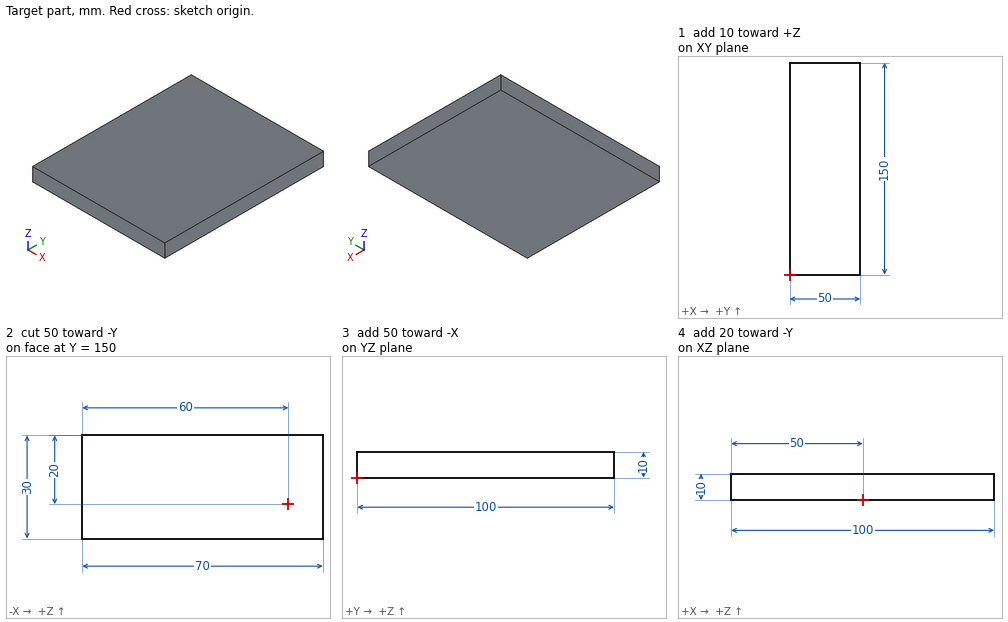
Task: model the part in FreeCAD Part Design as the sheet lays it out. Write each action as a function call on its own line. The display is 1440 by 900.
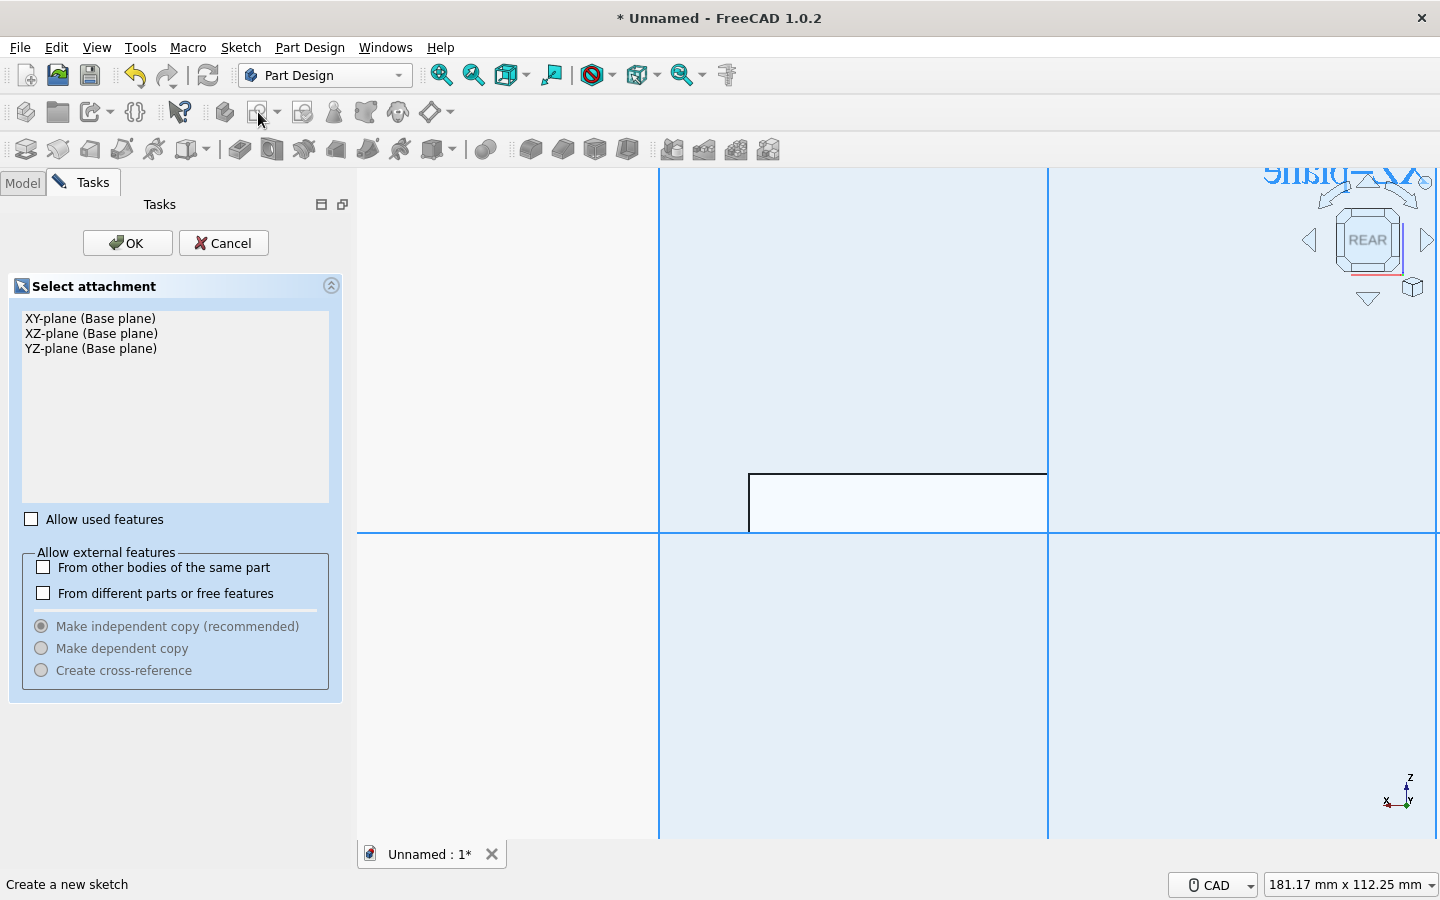
click(82, 348)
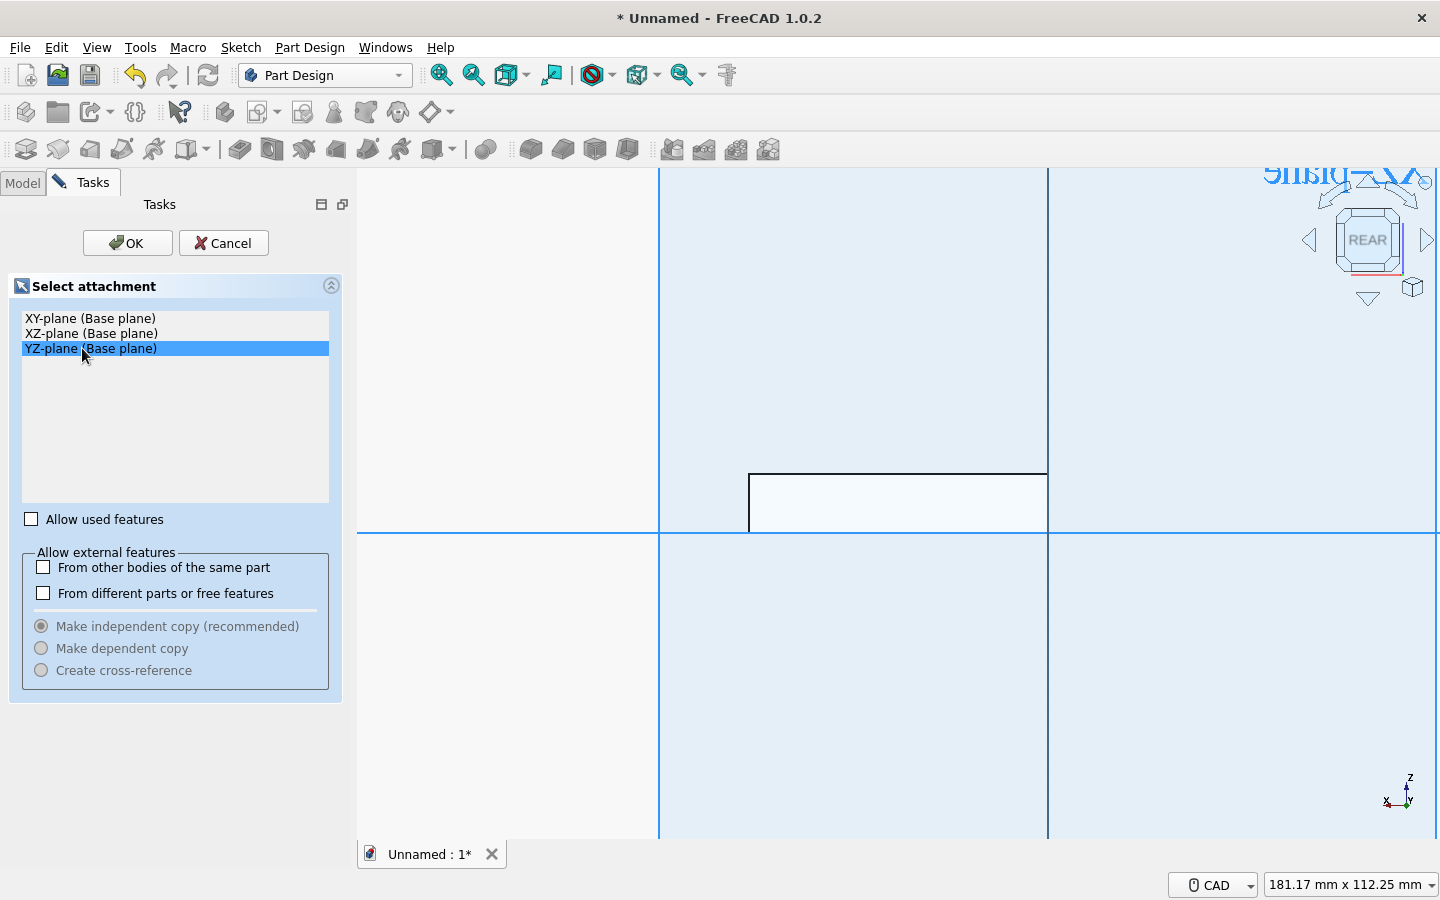
click(128, 243)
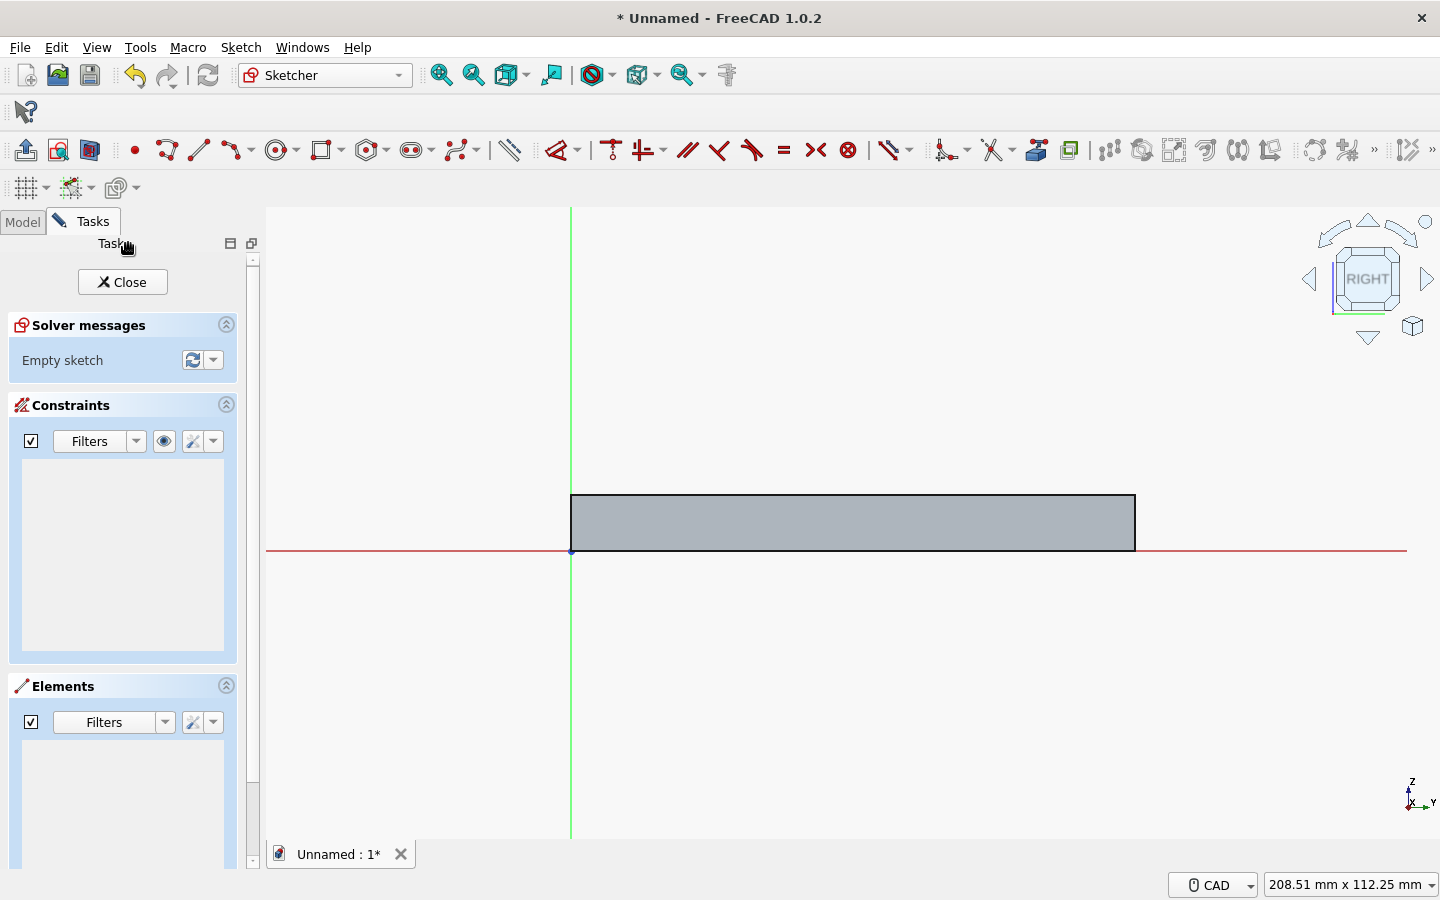
click(90, 150)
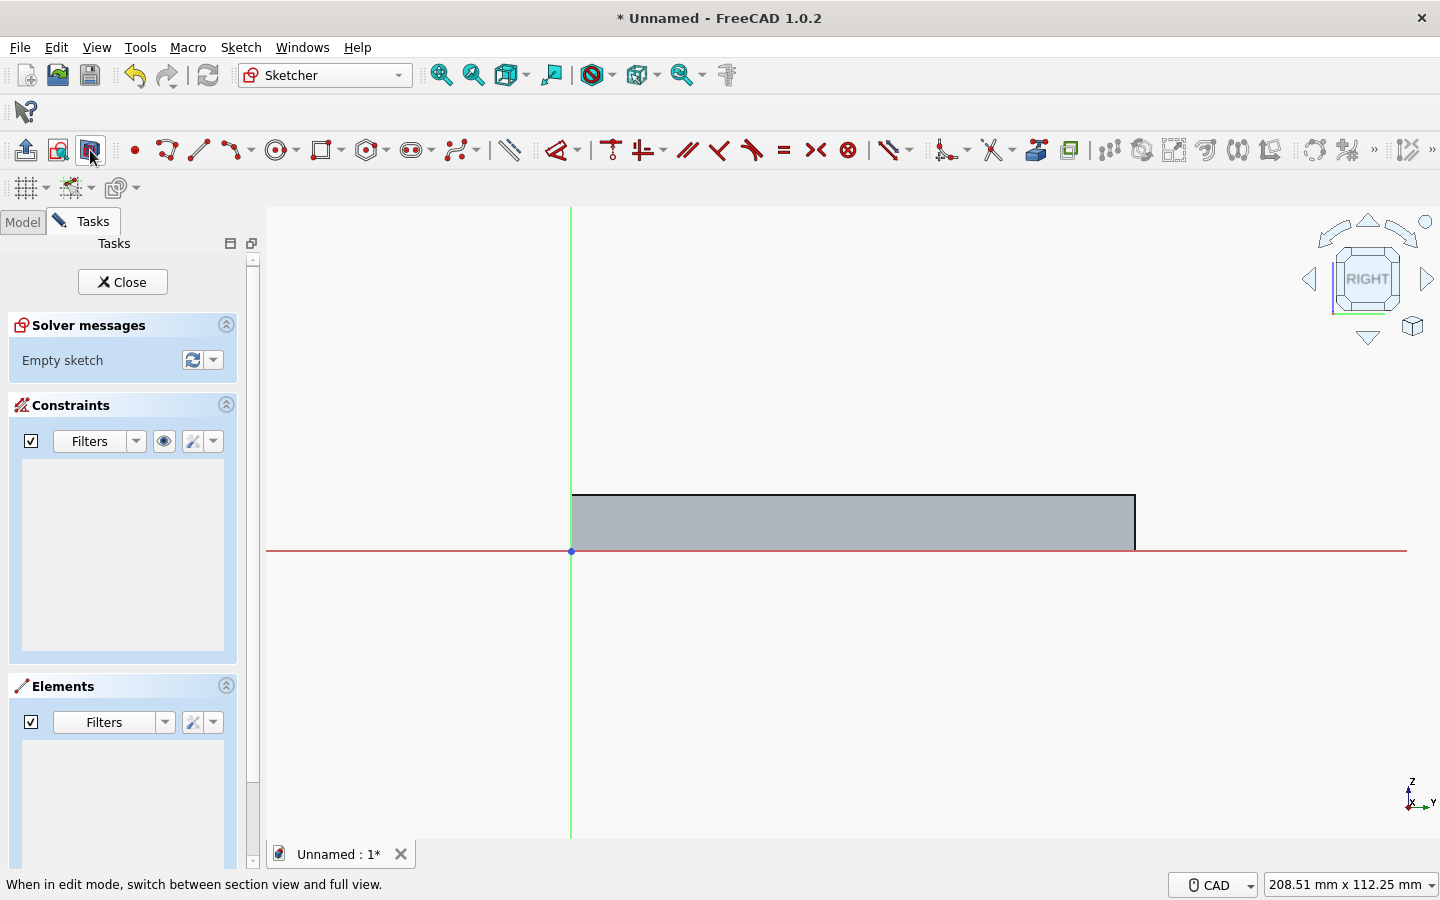
click(322, 150)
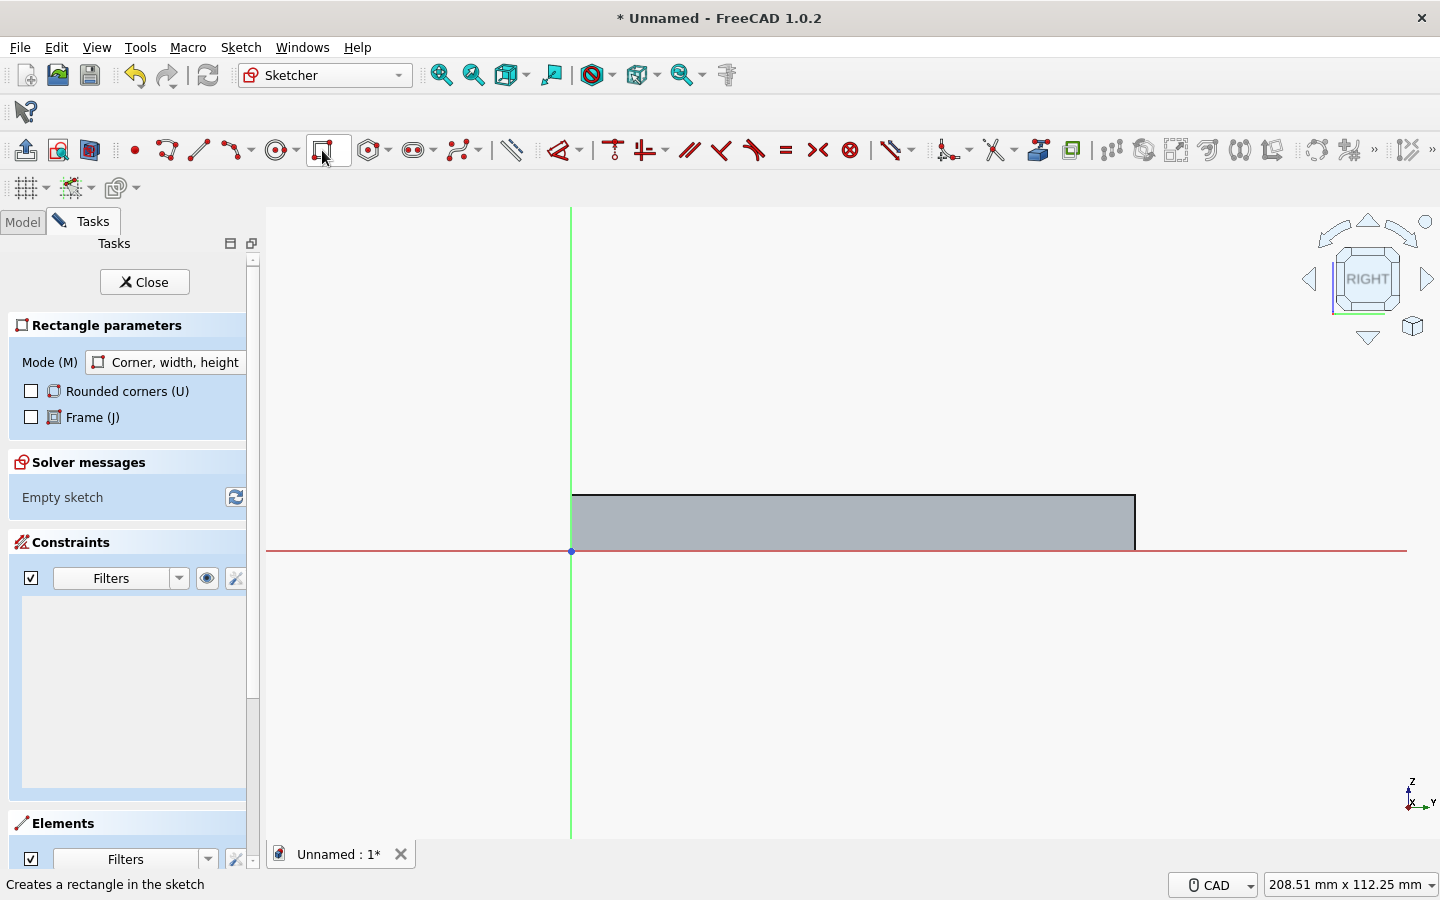
click(571, 551)
click(1135, 495)
key(Escape)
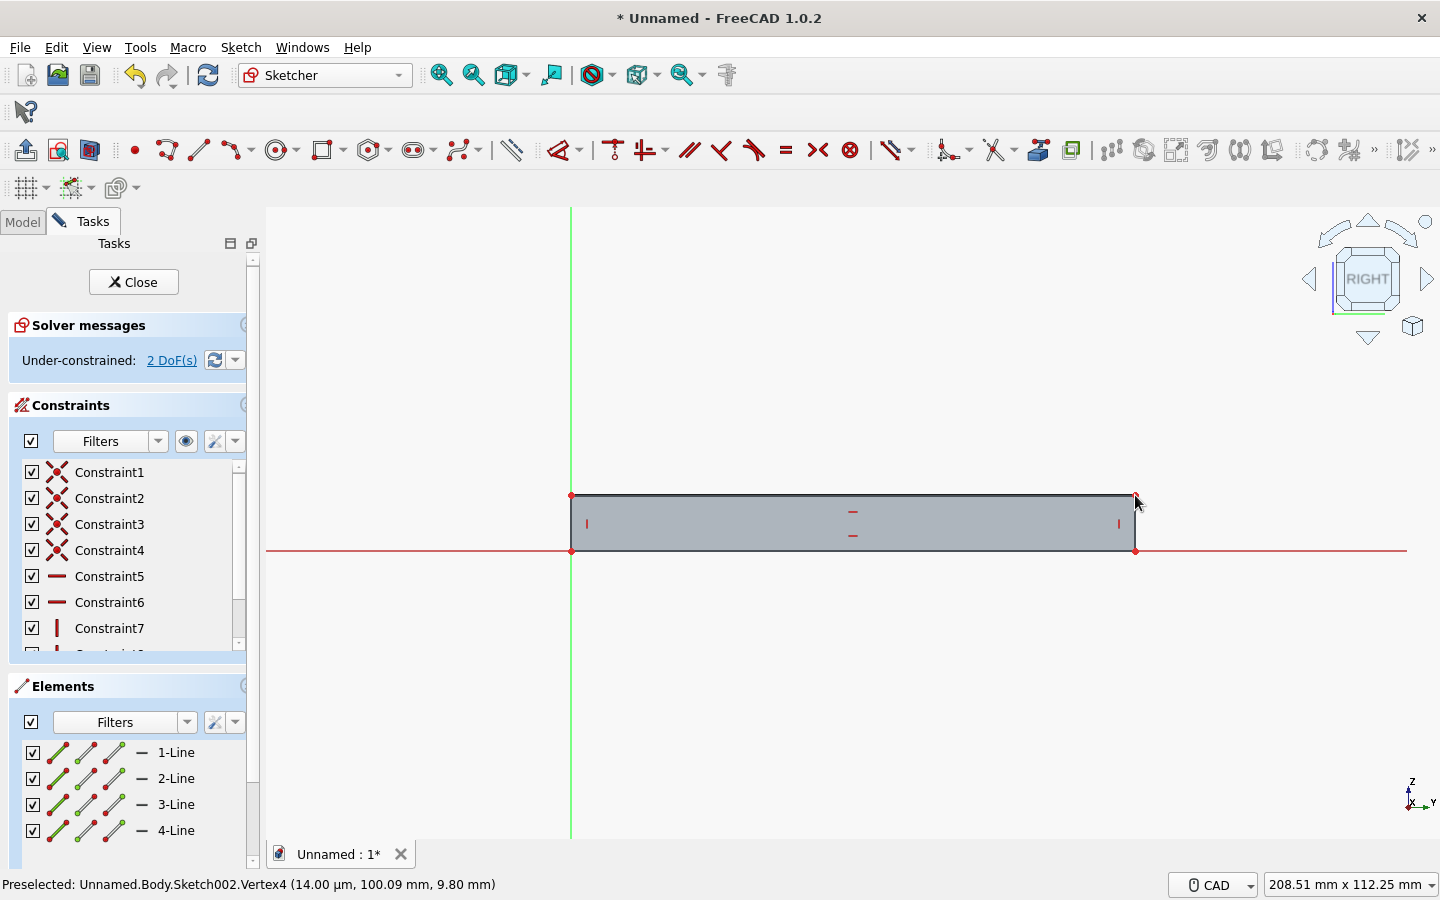
click(558, 150)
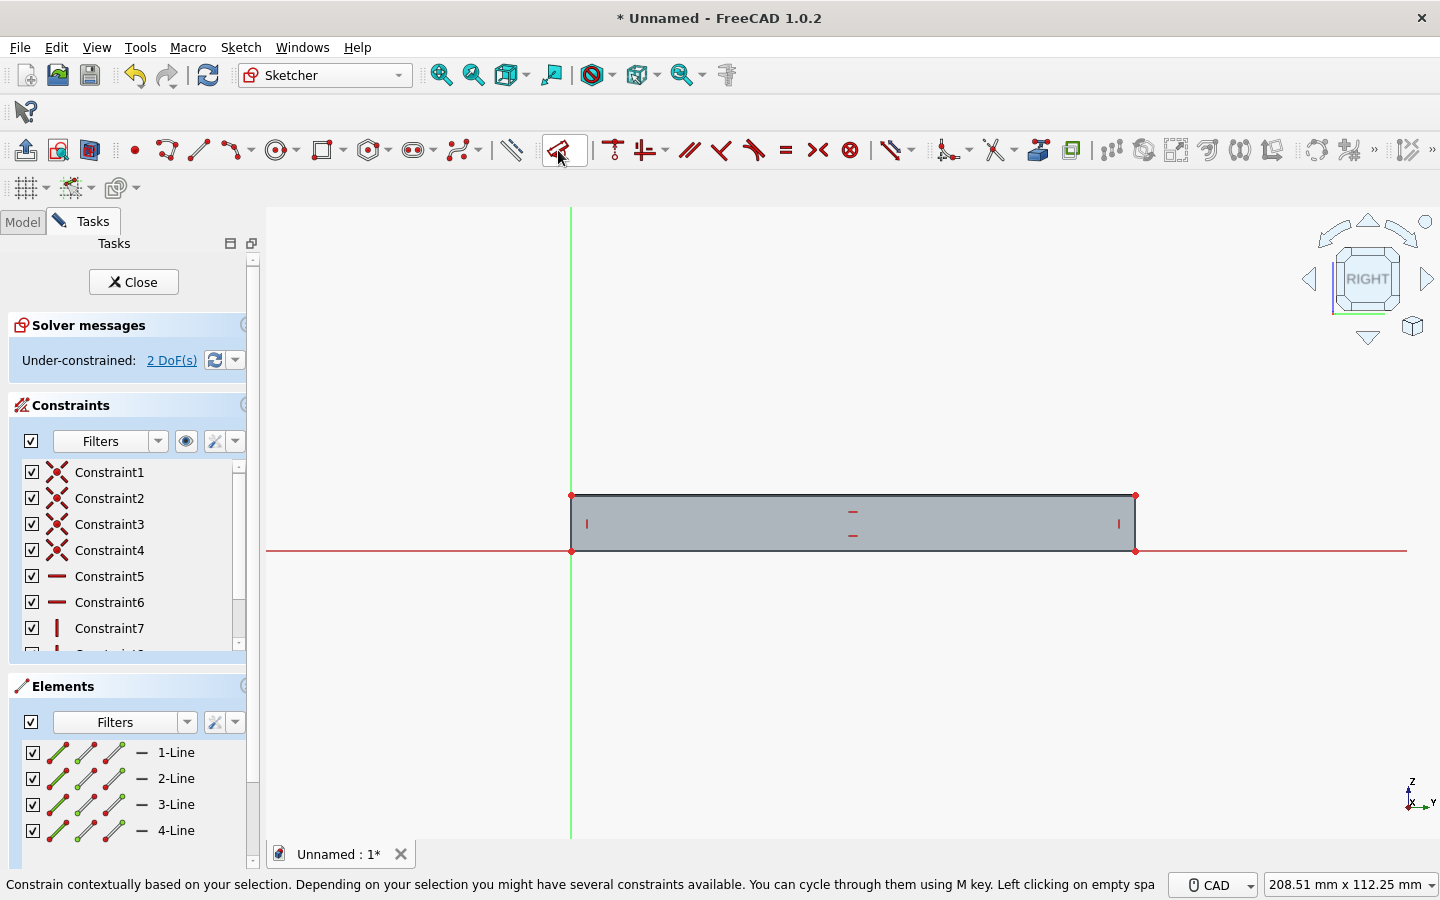
click(1135, 535)
click(1169, 524)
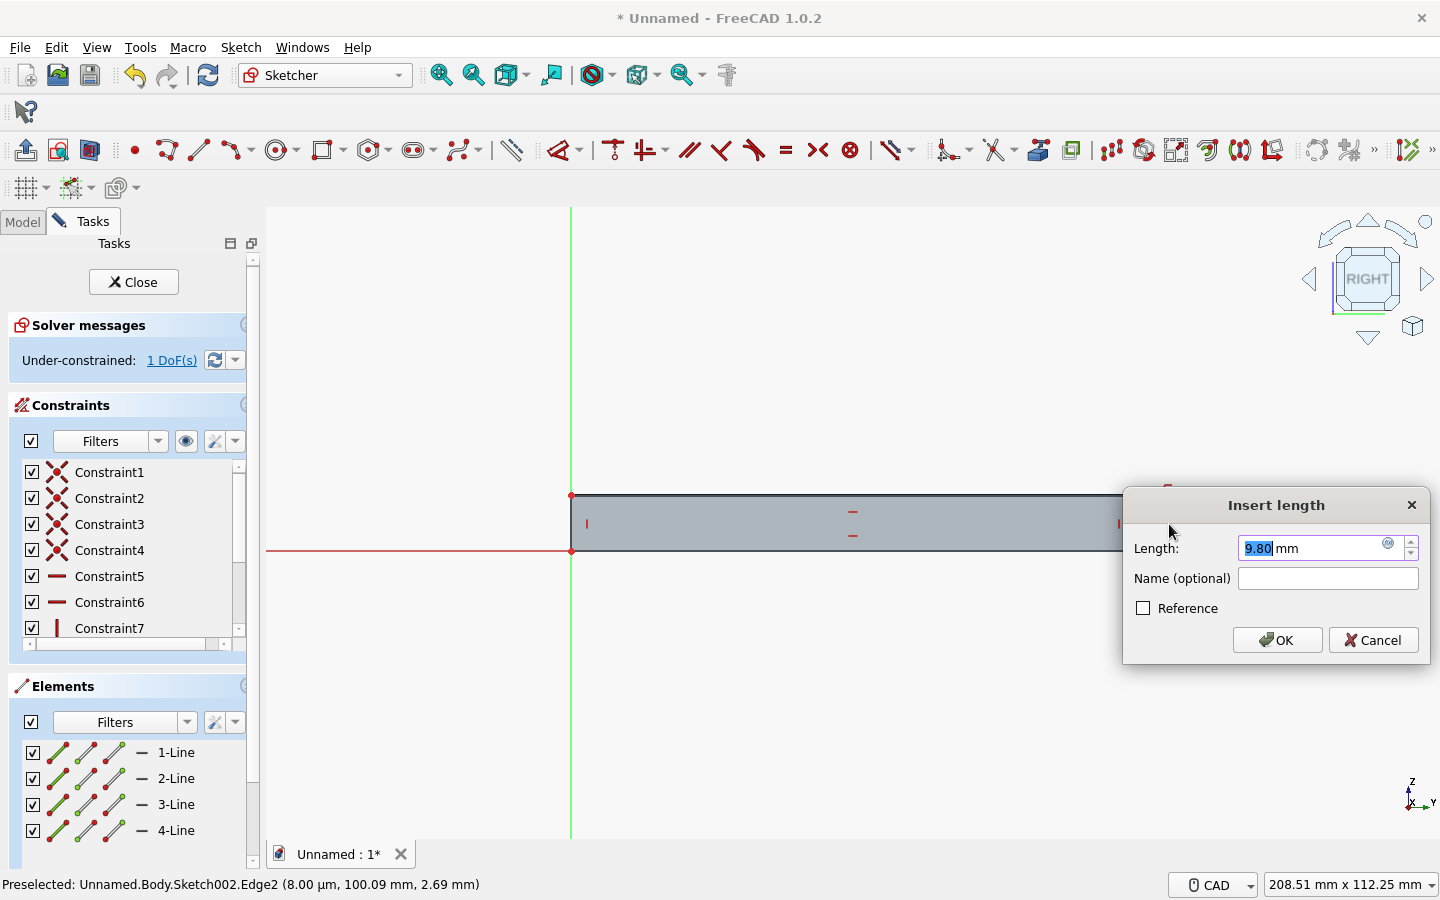
text(10)
key(Return)